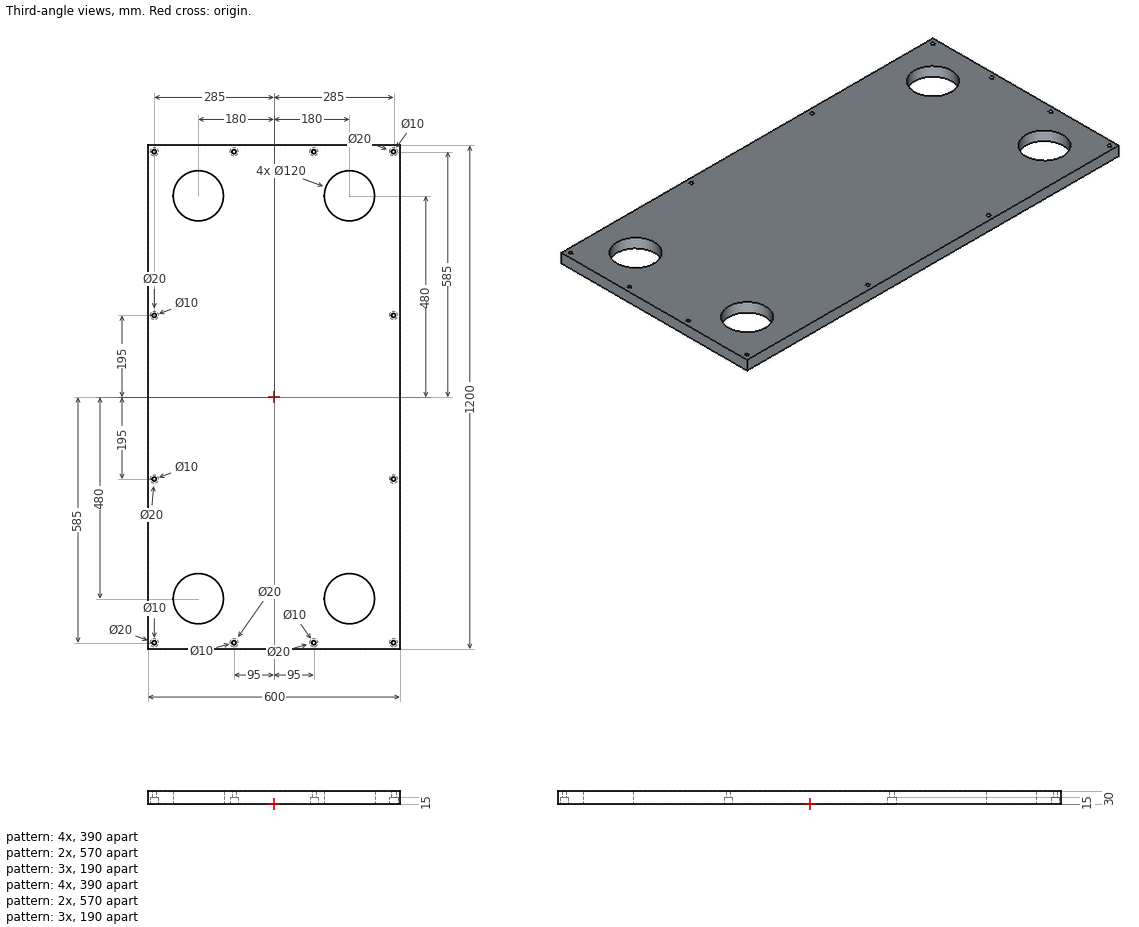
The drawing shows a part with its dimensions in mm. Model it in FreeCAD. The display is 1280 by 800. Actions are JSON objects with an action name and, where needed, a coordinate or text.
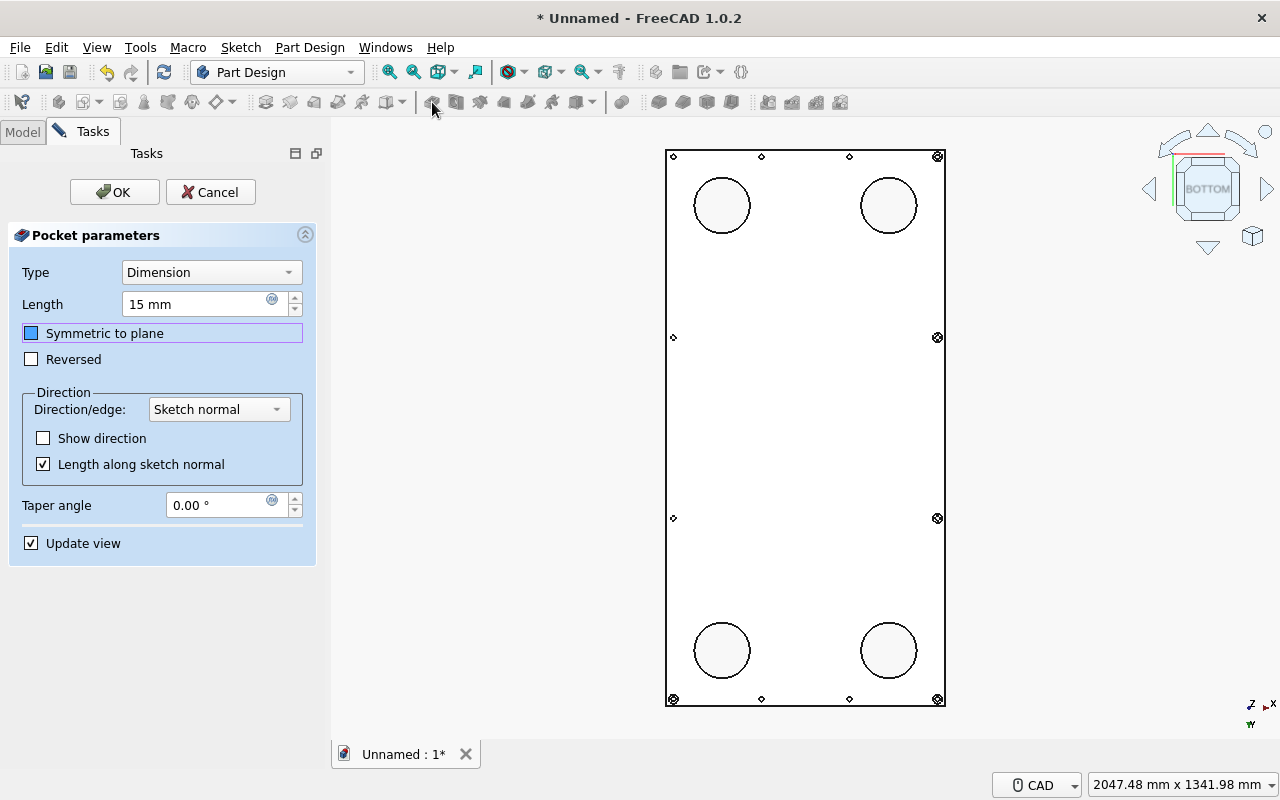
{"action": "left_click", "coordinate": [30, 359]}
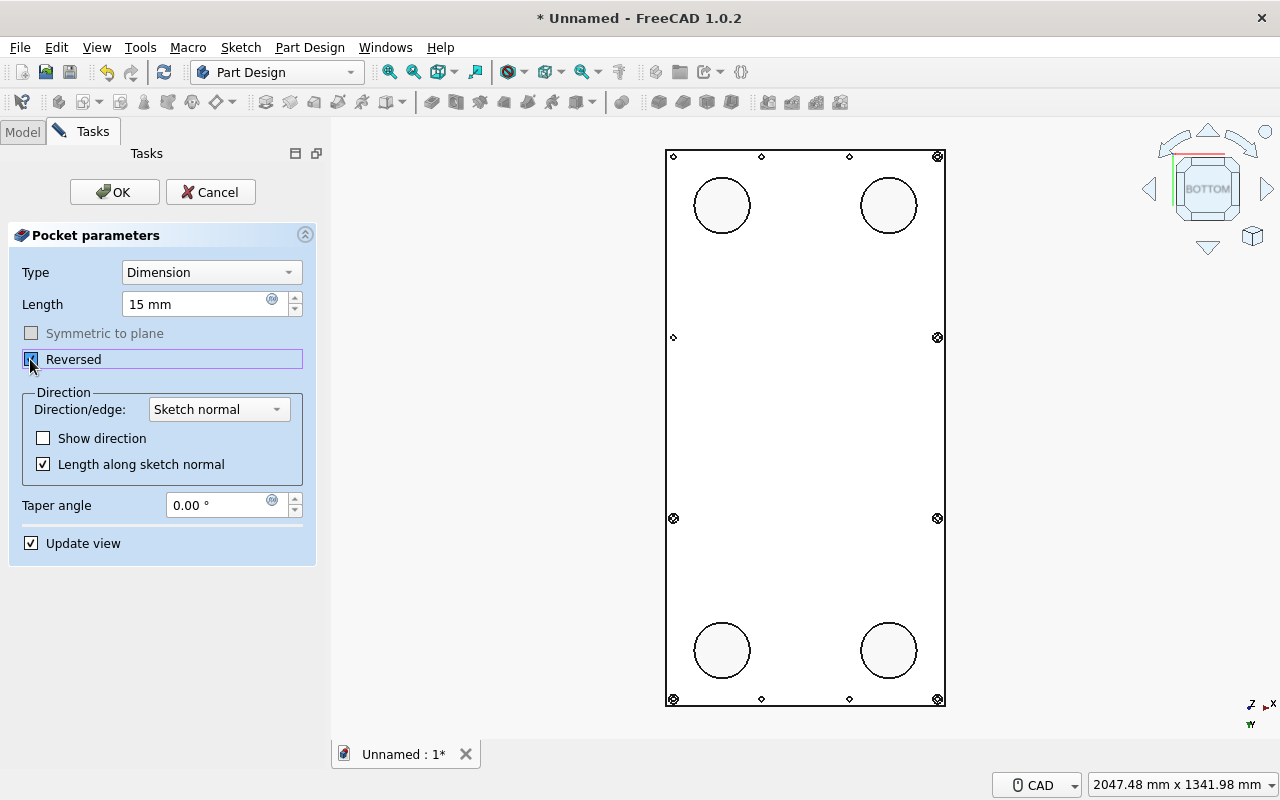
{"action": "left_click", "coordinate": [115, 192]}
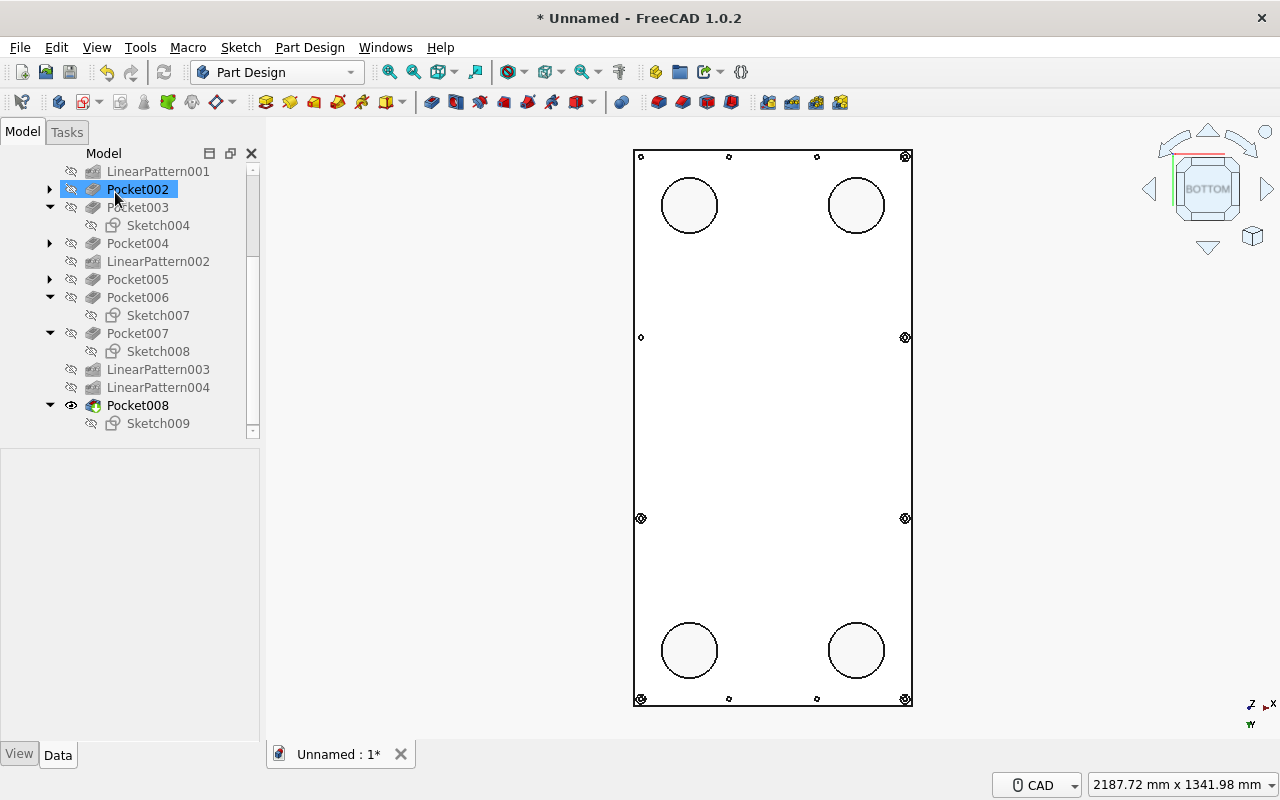
{"action": "left_click", "coordinate": [84, 102]}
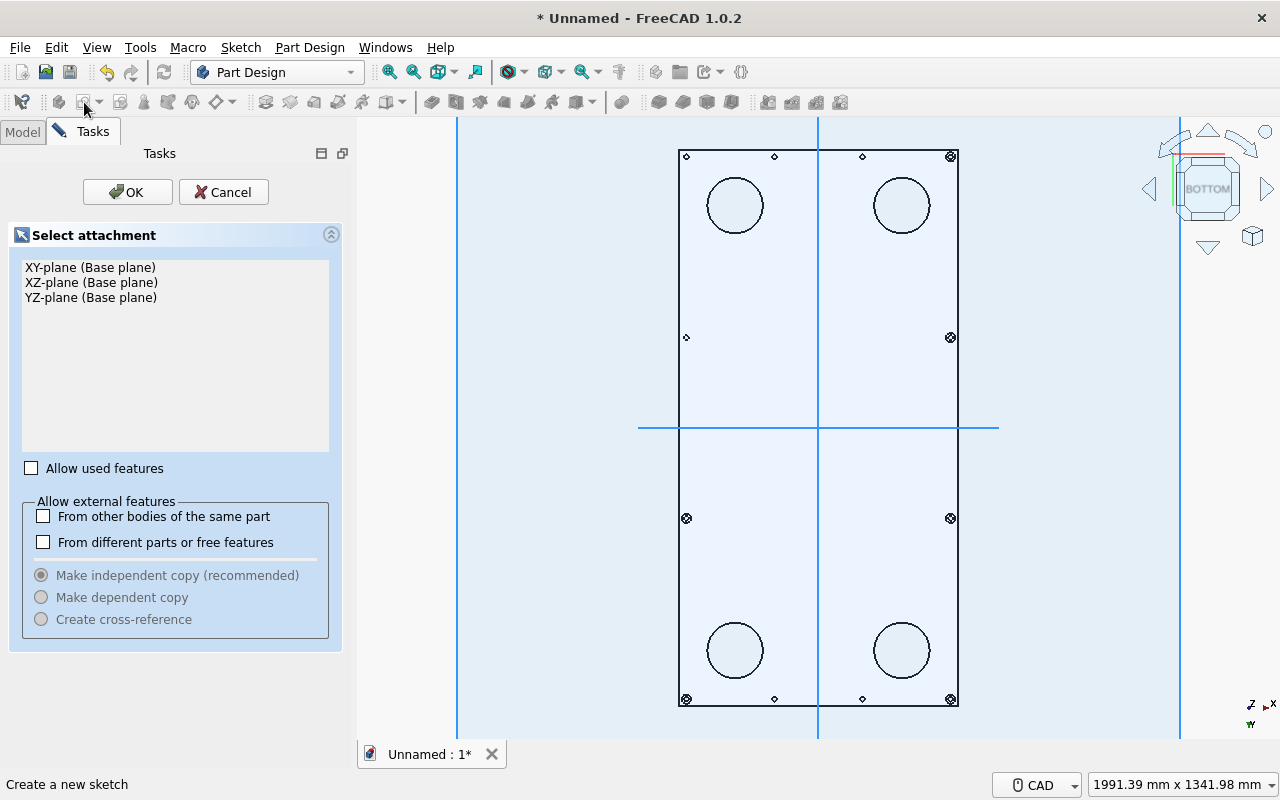
{"action": "left_click", "coordinate": [82, 268]}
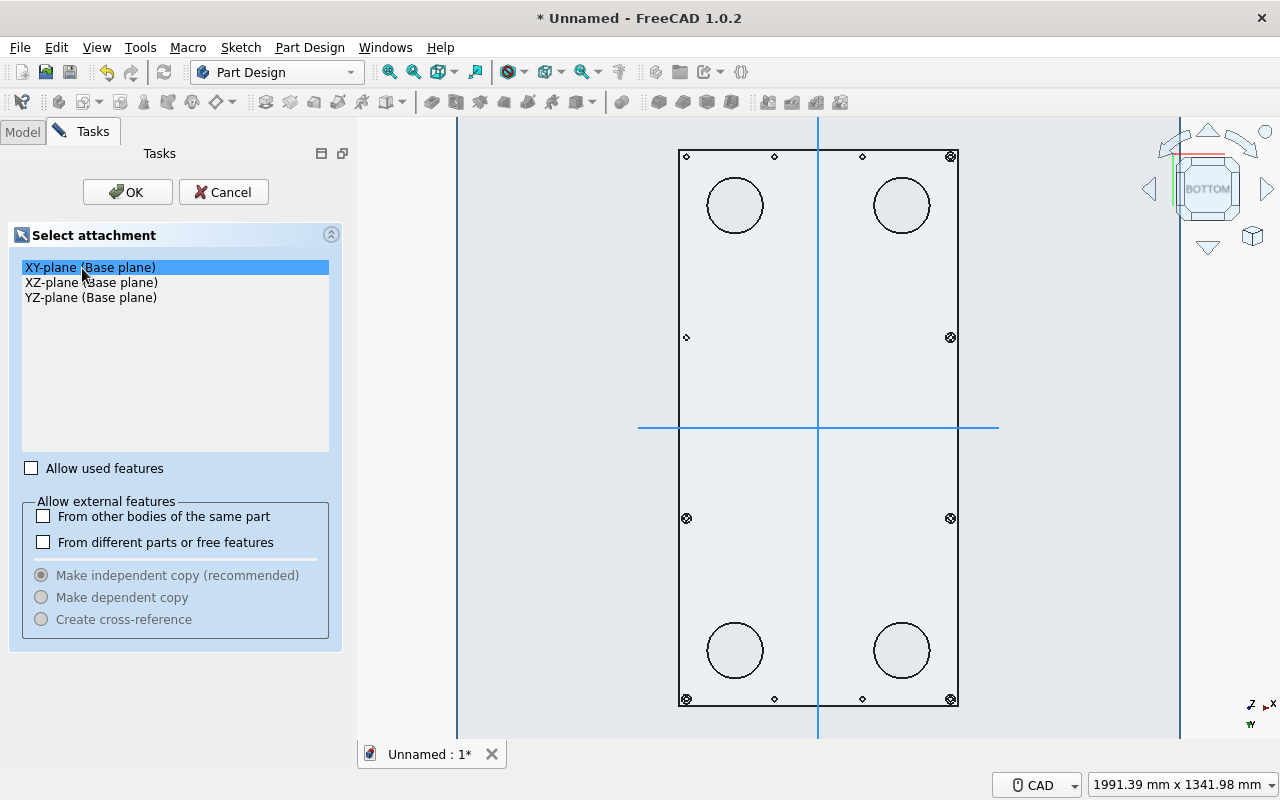
{"action": "left_click", "coordinate": [128, 192]}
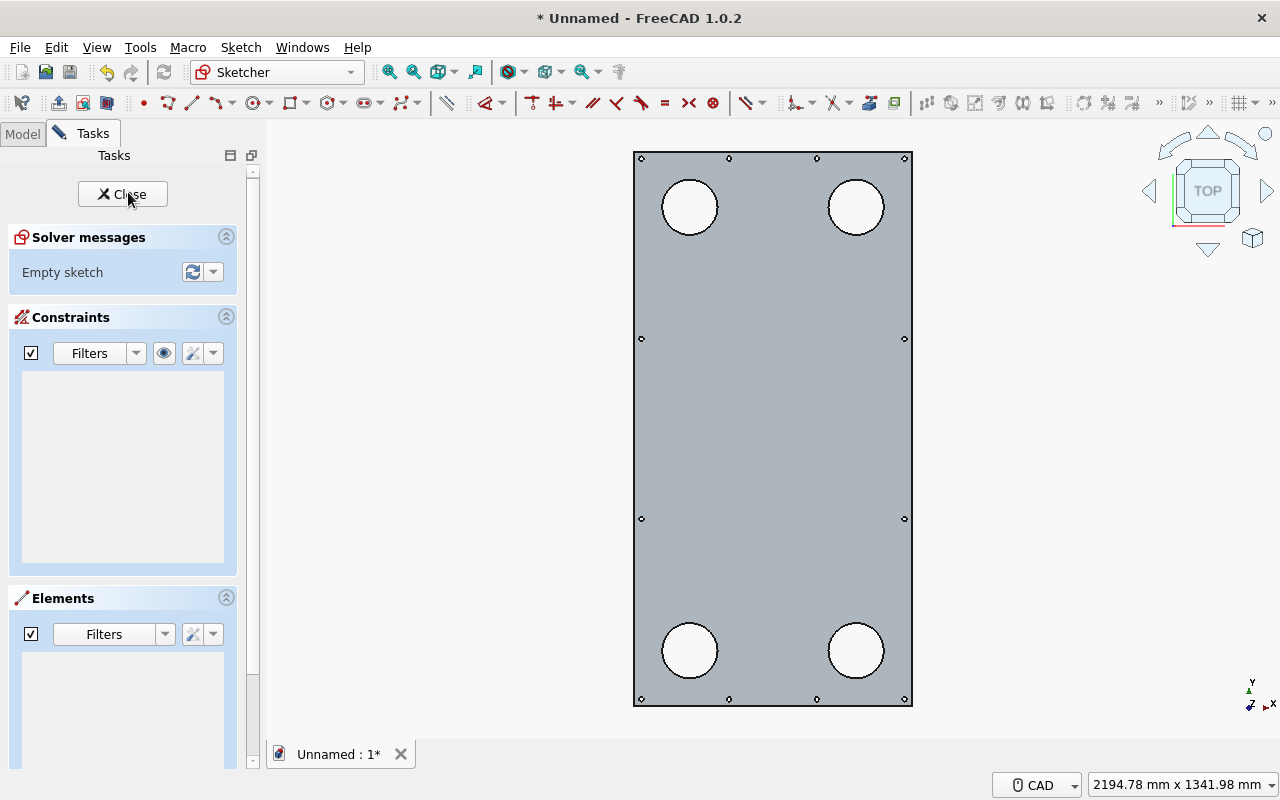
{"action": "left_click", "coordinate": [108, 104]}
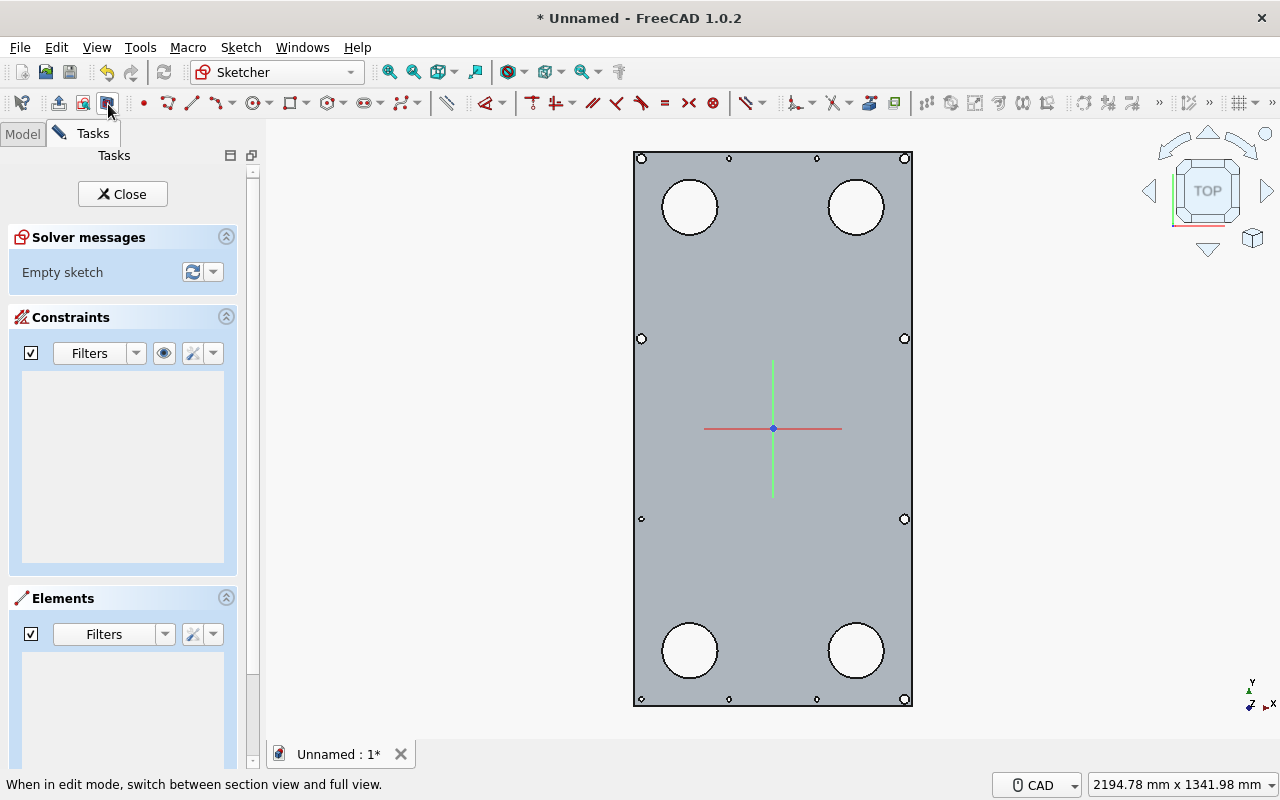
{"action": "scroll", "coordinate": [638, 524], "scroll_direction": "up", "scroll_amount": 15}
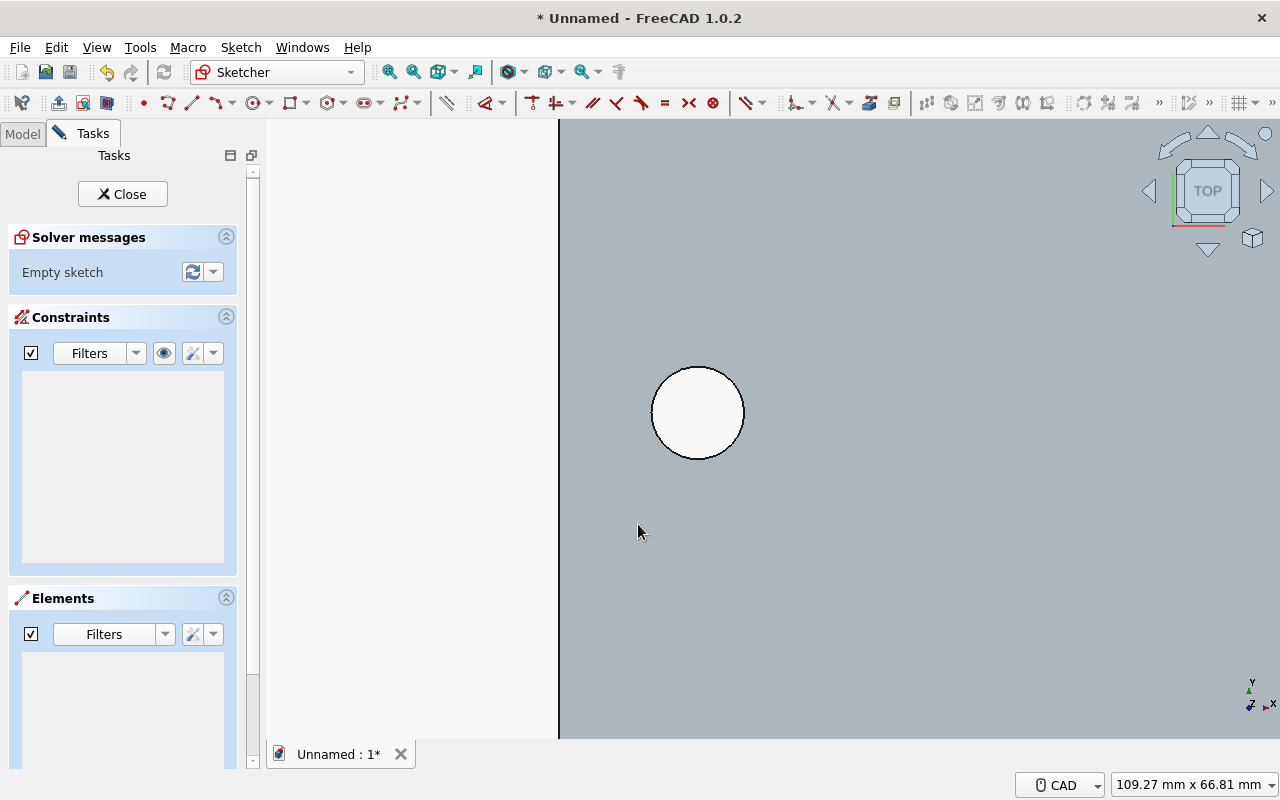
{"action": "scroll", "coordinate": [692, 400], "scroll_direction": "up", "scroll_amount": 4}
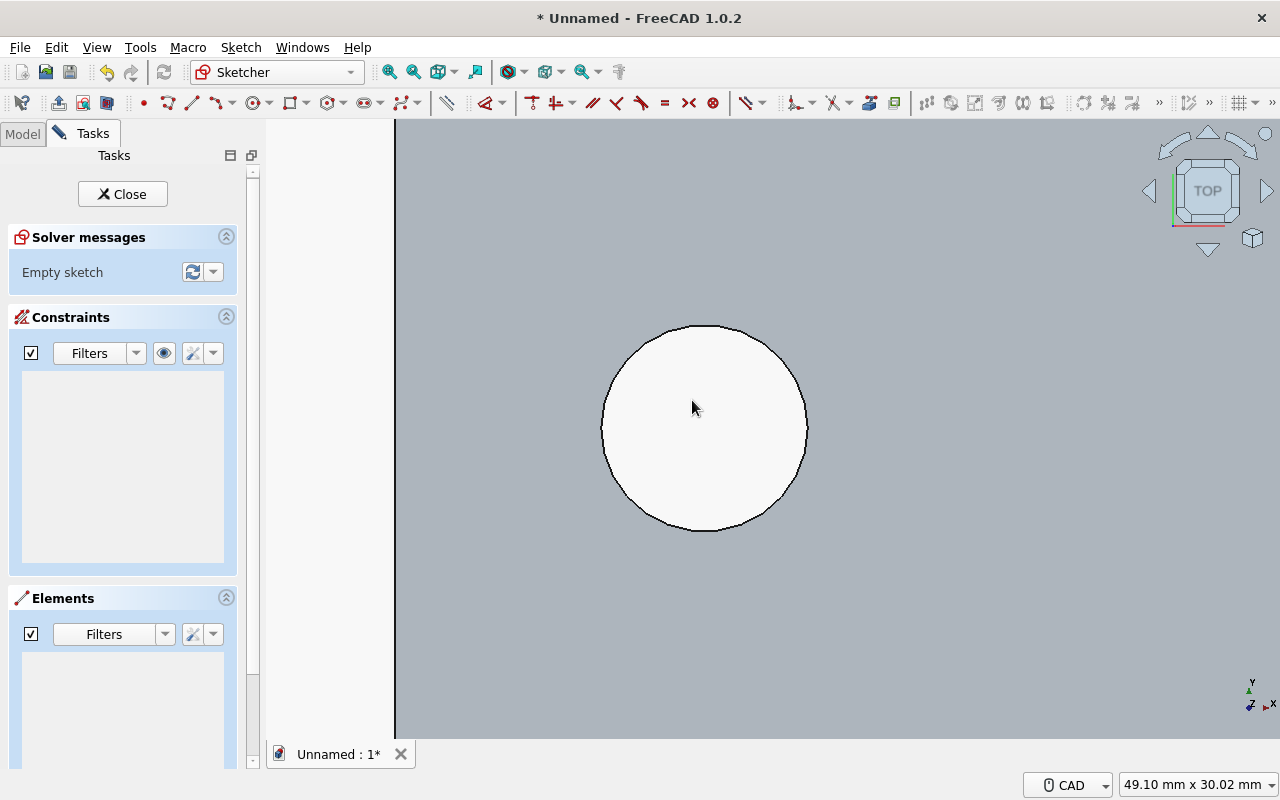
{"action": "key", "text": "g c"}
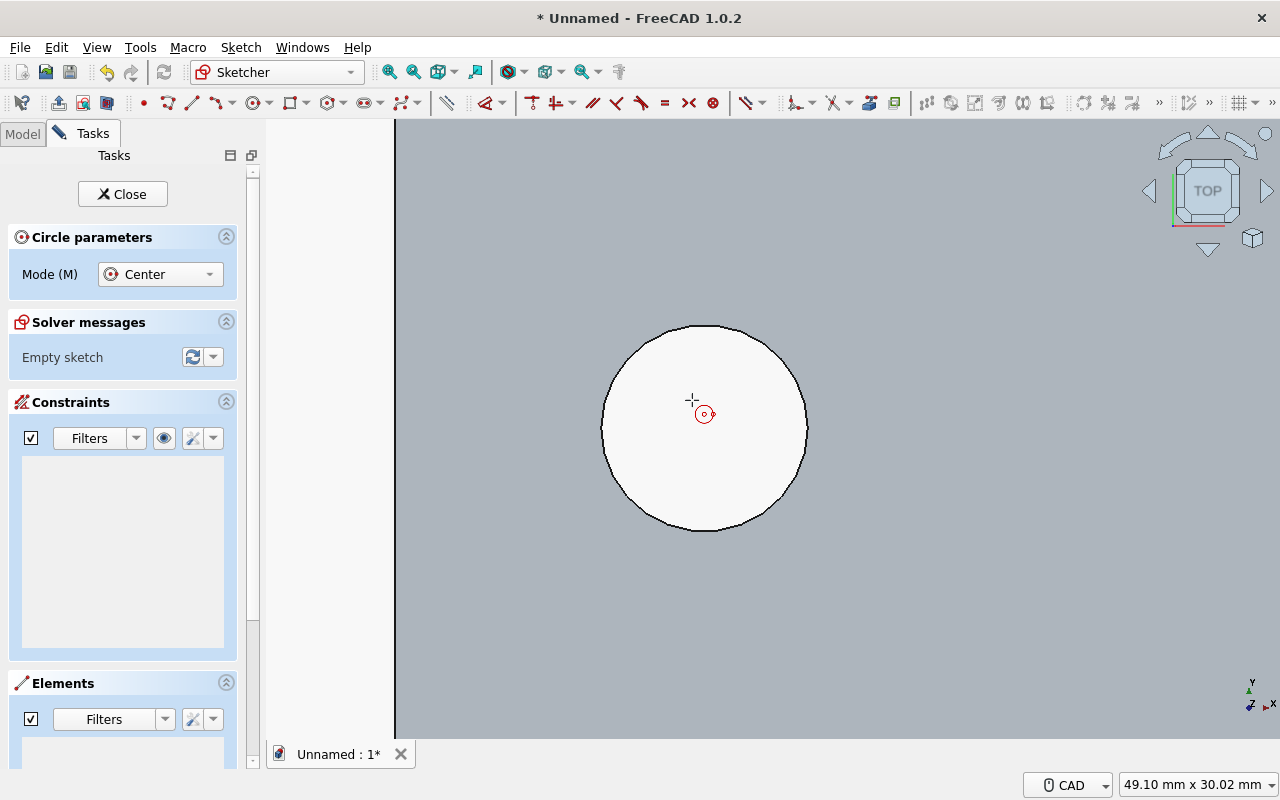
{"action": "left_click", "coordinate": [704, 428]}
{"action": "mouse_move", "coordinate": [851, 282]}